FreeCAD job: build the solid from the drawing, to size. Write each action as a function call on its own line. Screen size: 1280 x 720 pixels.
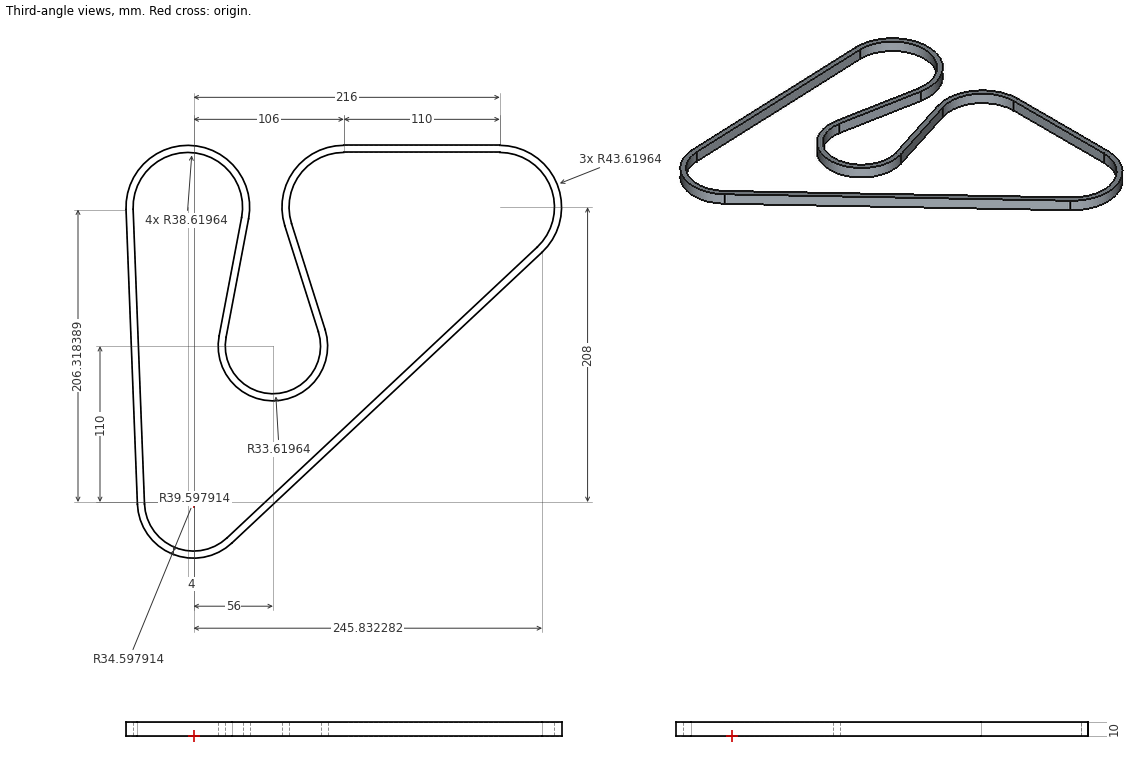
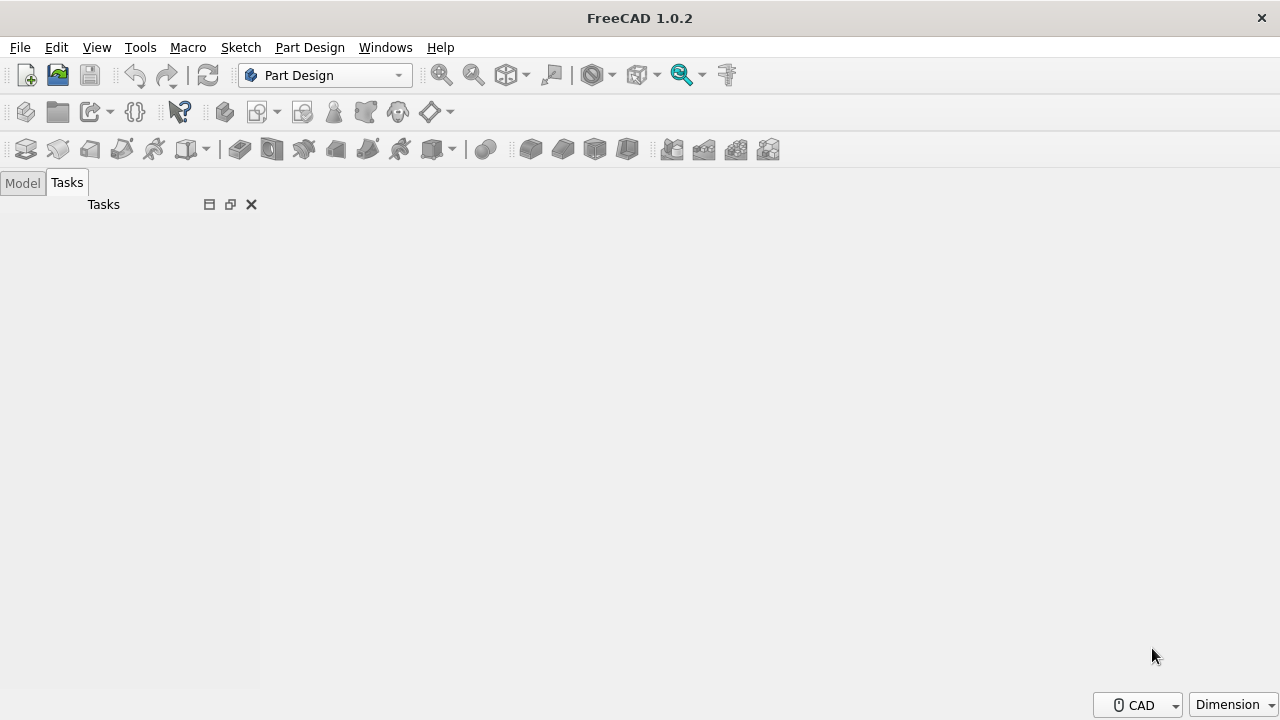
click(26, 76)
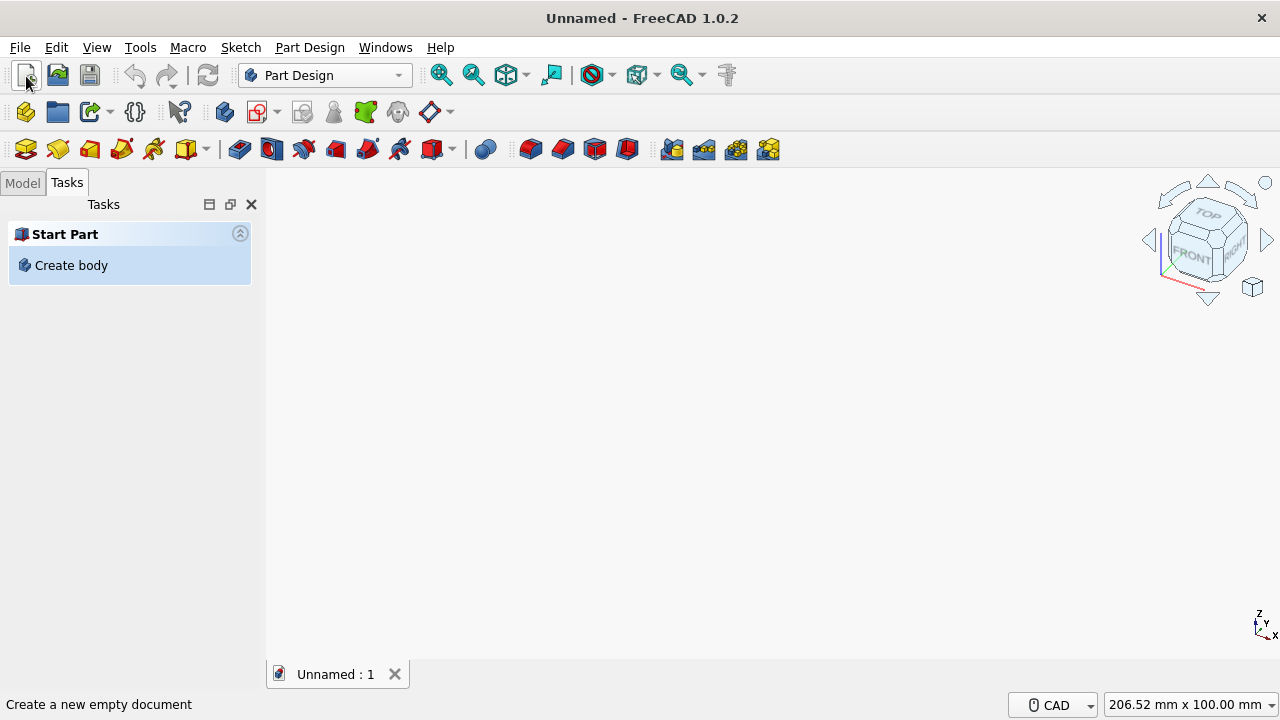
click(258, 112)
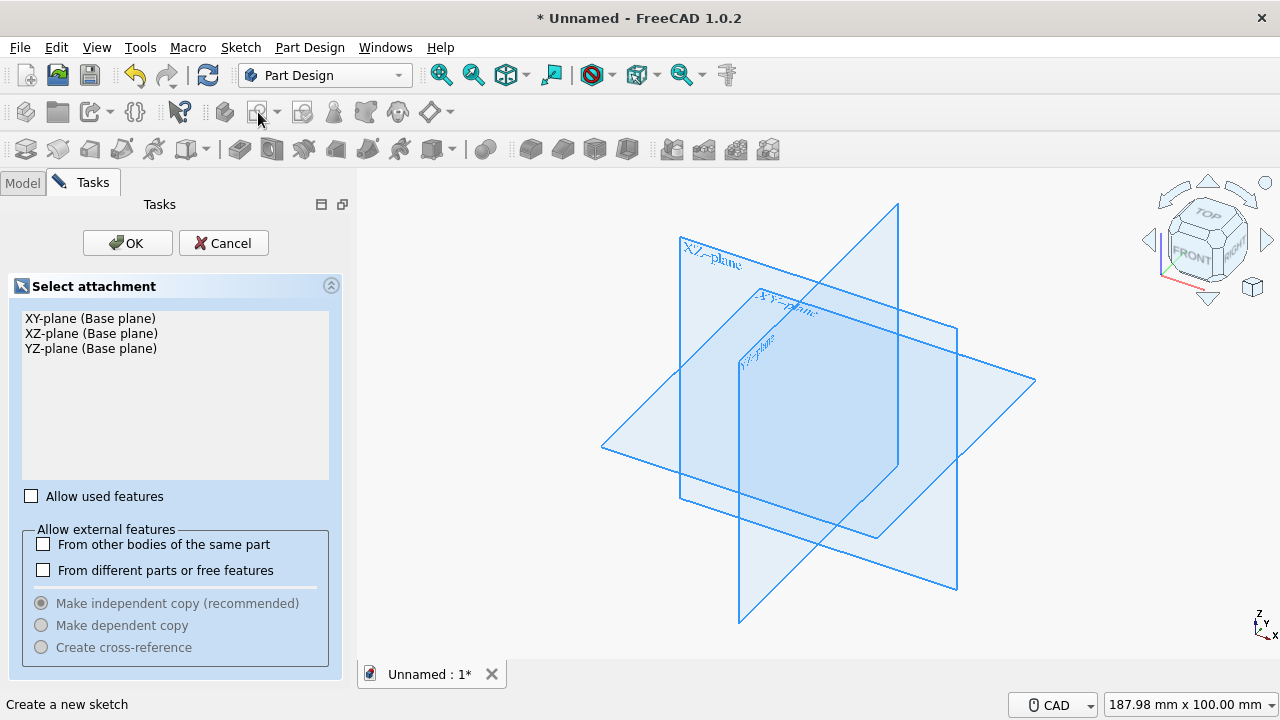
click(82, 318)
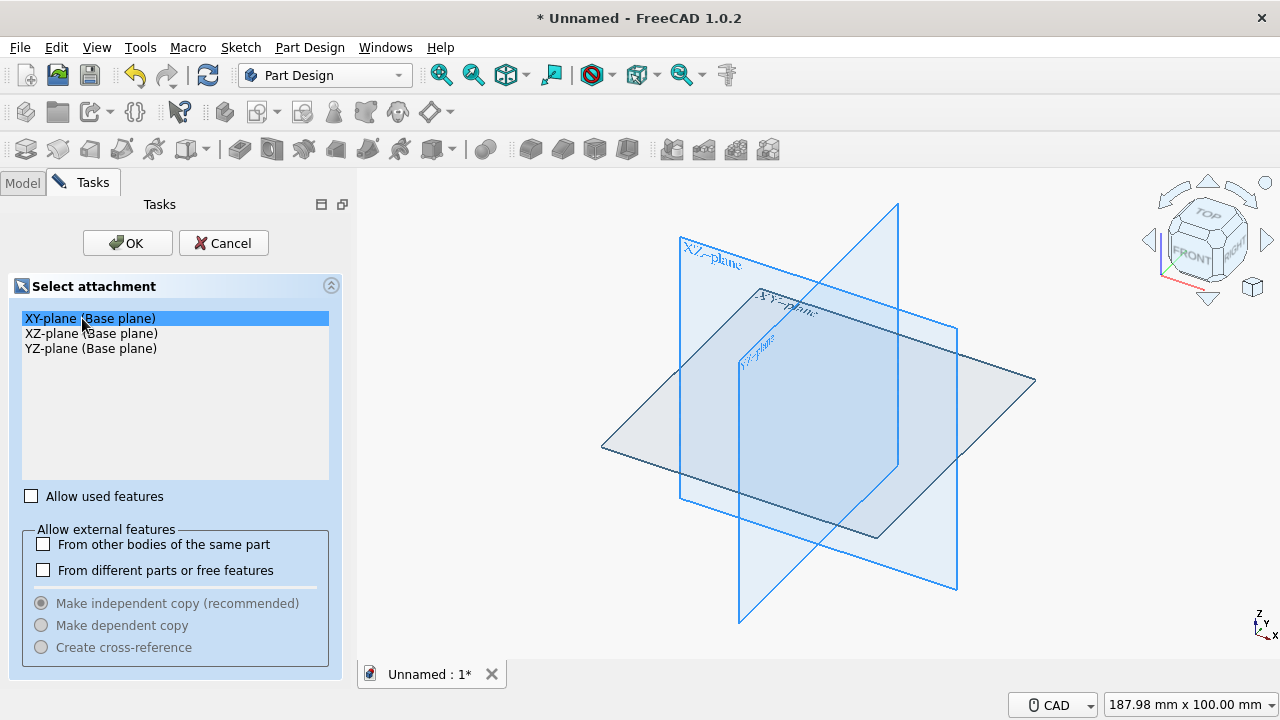
click(128, 243)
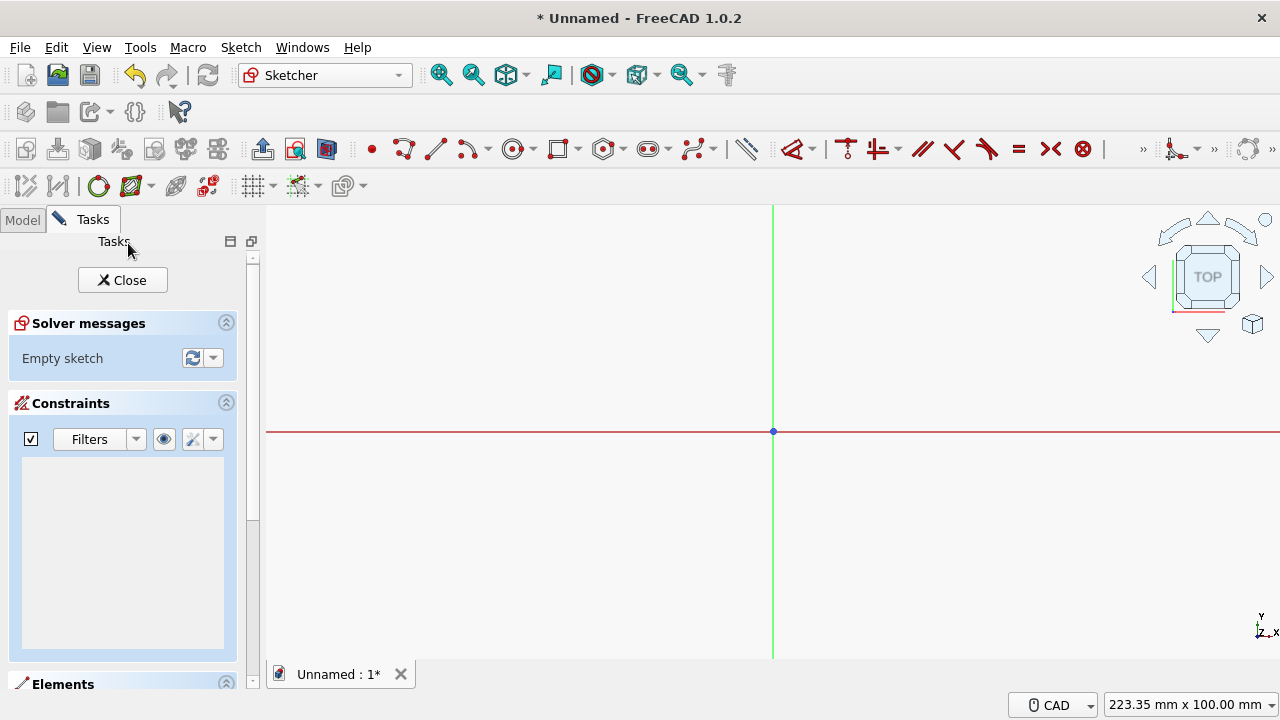
scroll(567, 555, down, 8)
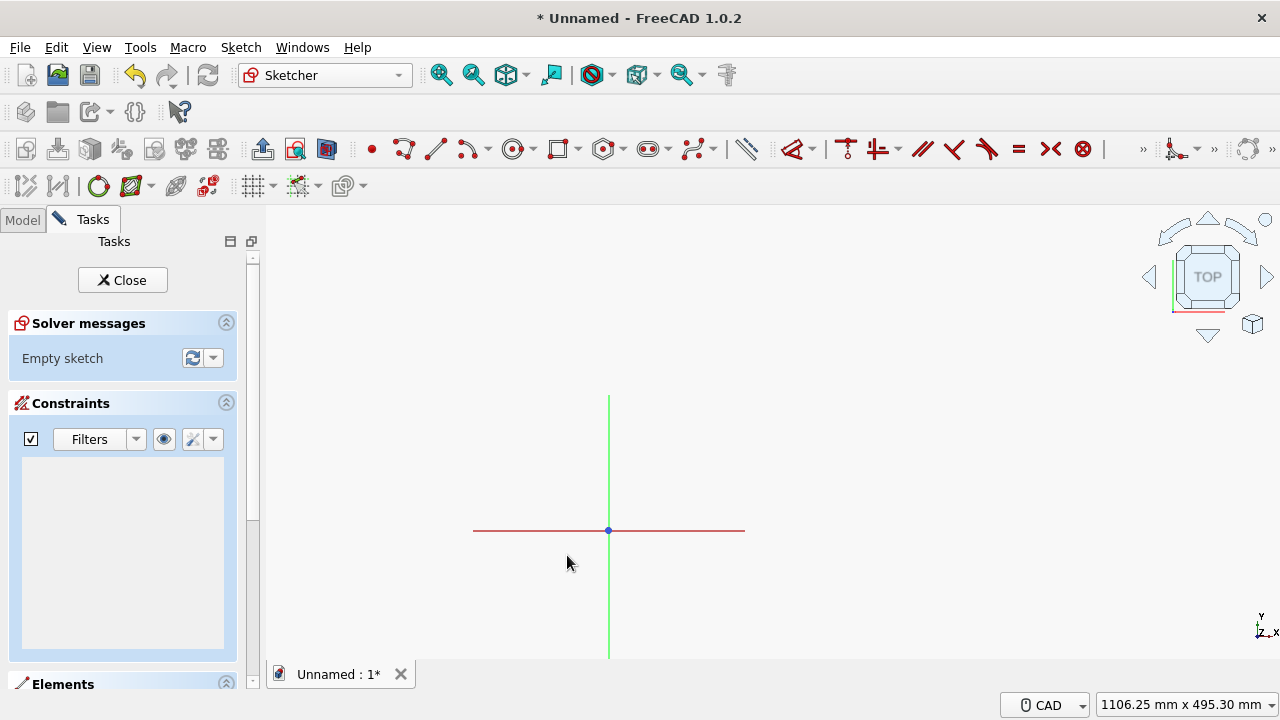
key(g)
key(l)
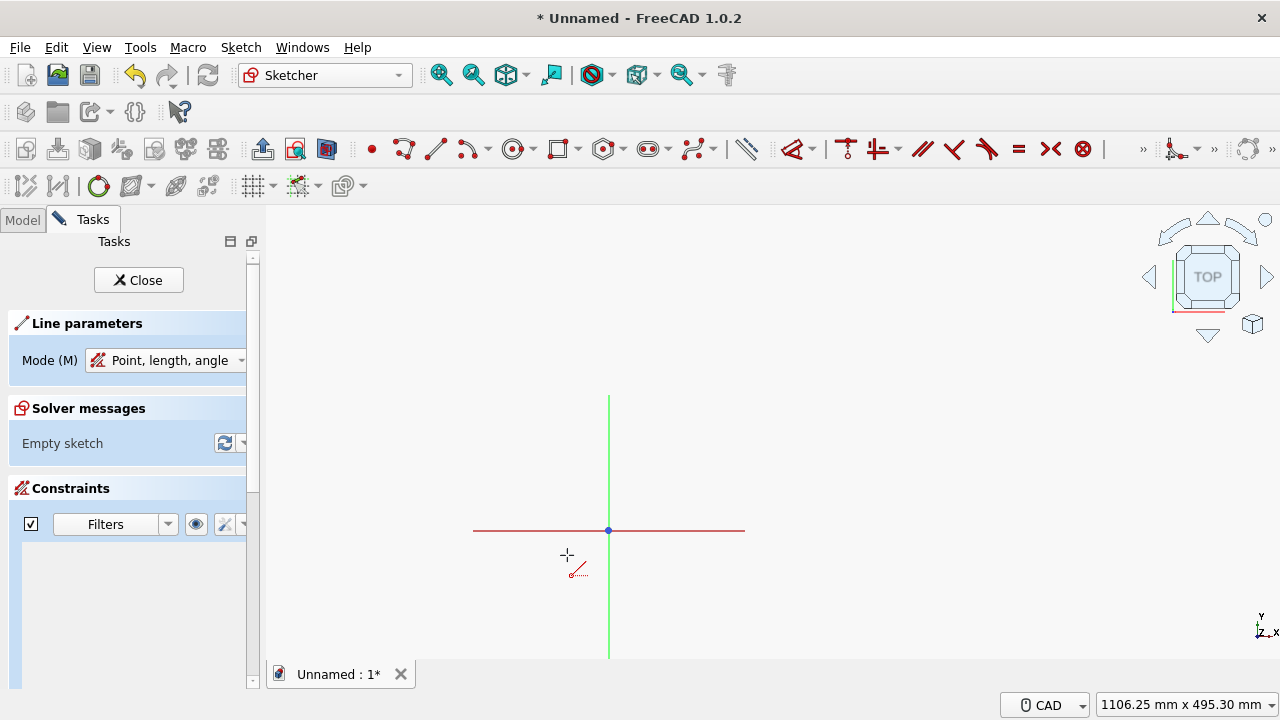
click(634, 557)
click(834, 369)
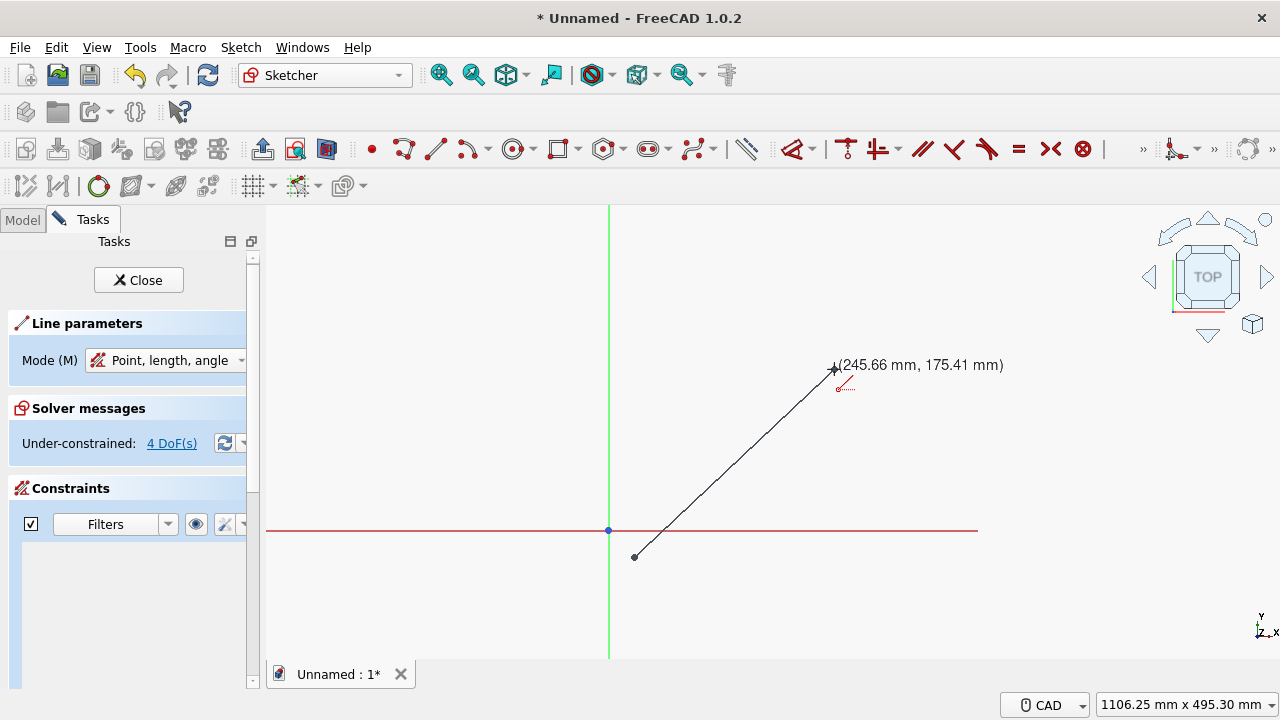
click(807, 300)
click(706, 300)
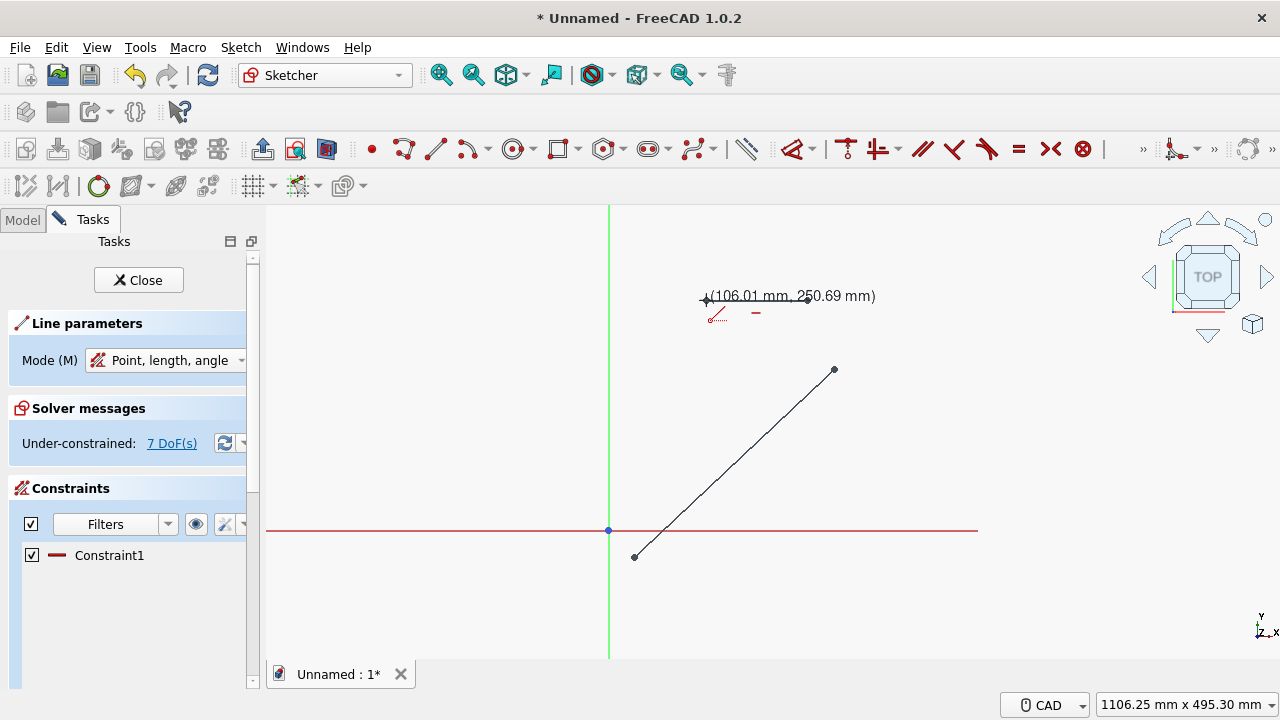
click(668, 352)
click(690, 421)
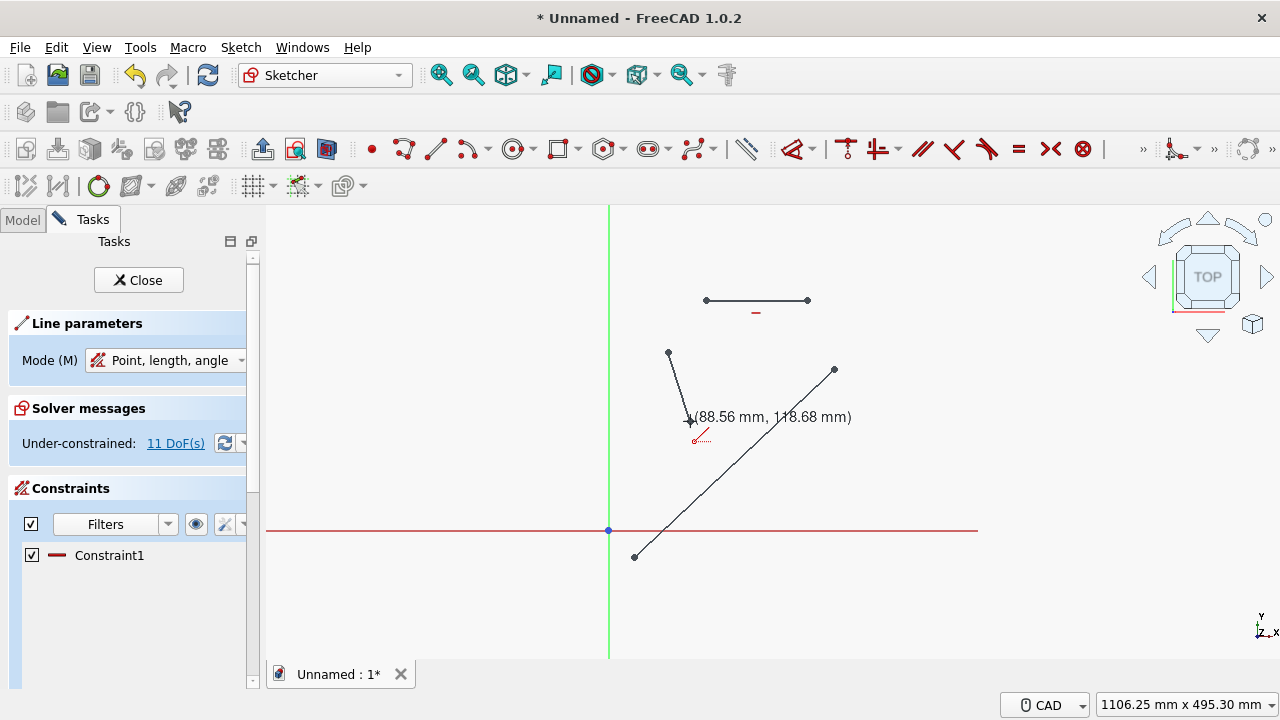
click(630, 424)
click(644, 348)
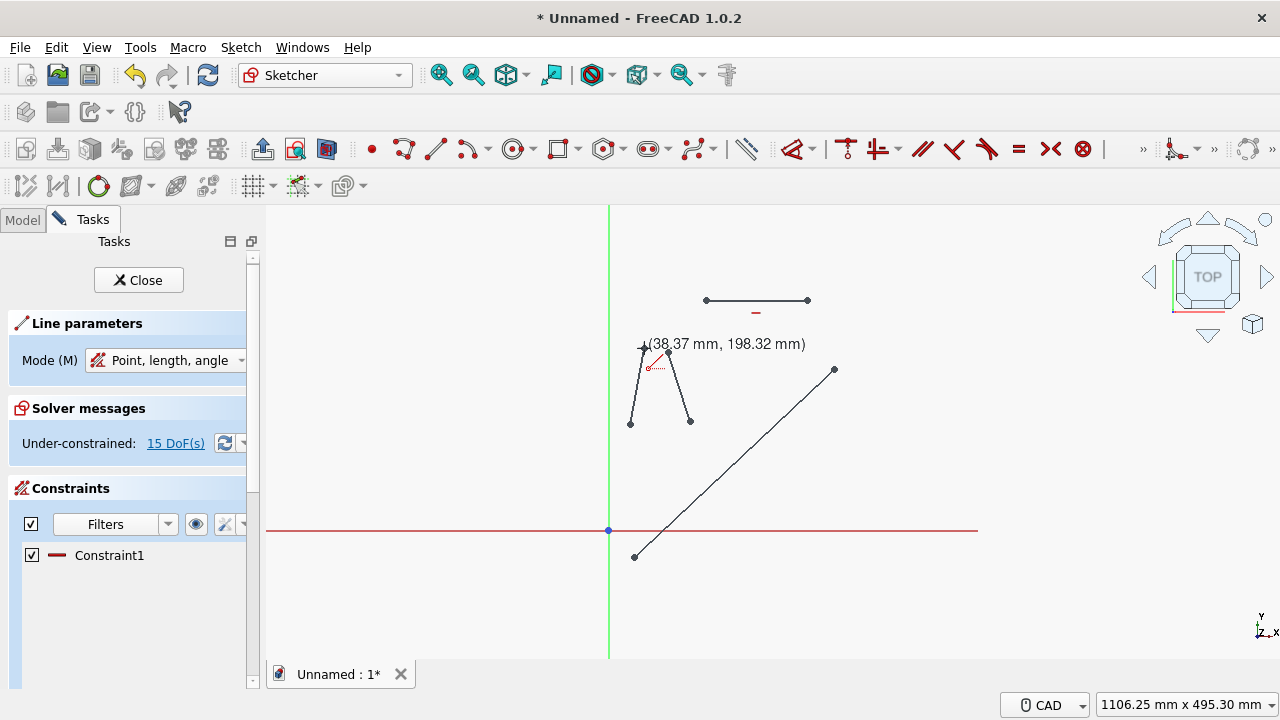
click(565, 342)